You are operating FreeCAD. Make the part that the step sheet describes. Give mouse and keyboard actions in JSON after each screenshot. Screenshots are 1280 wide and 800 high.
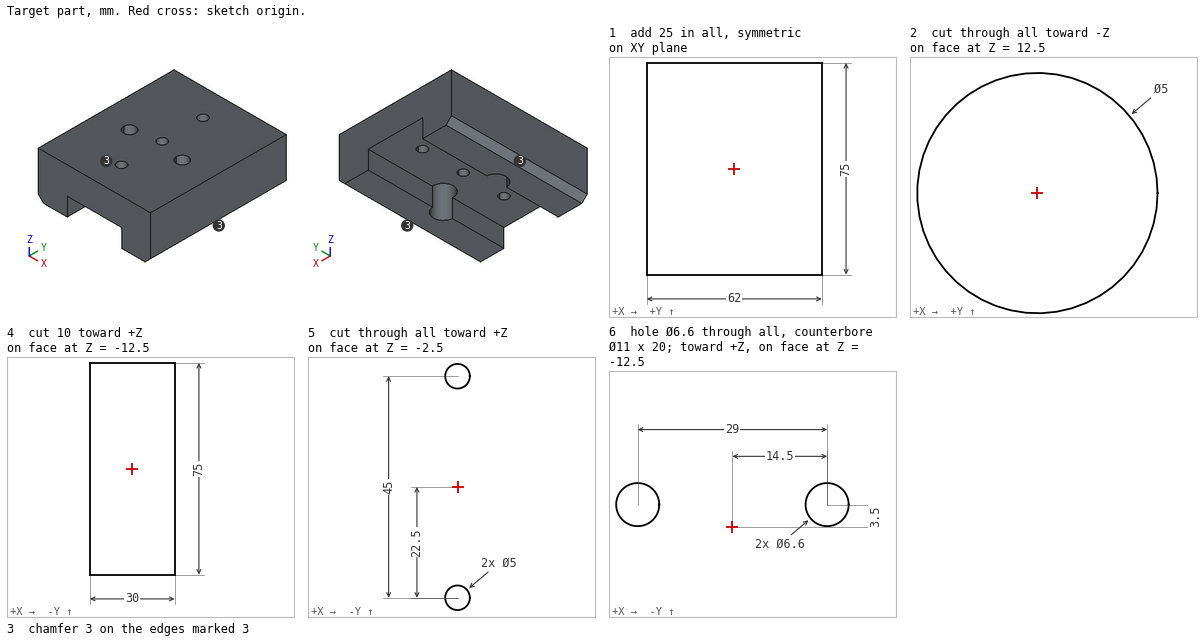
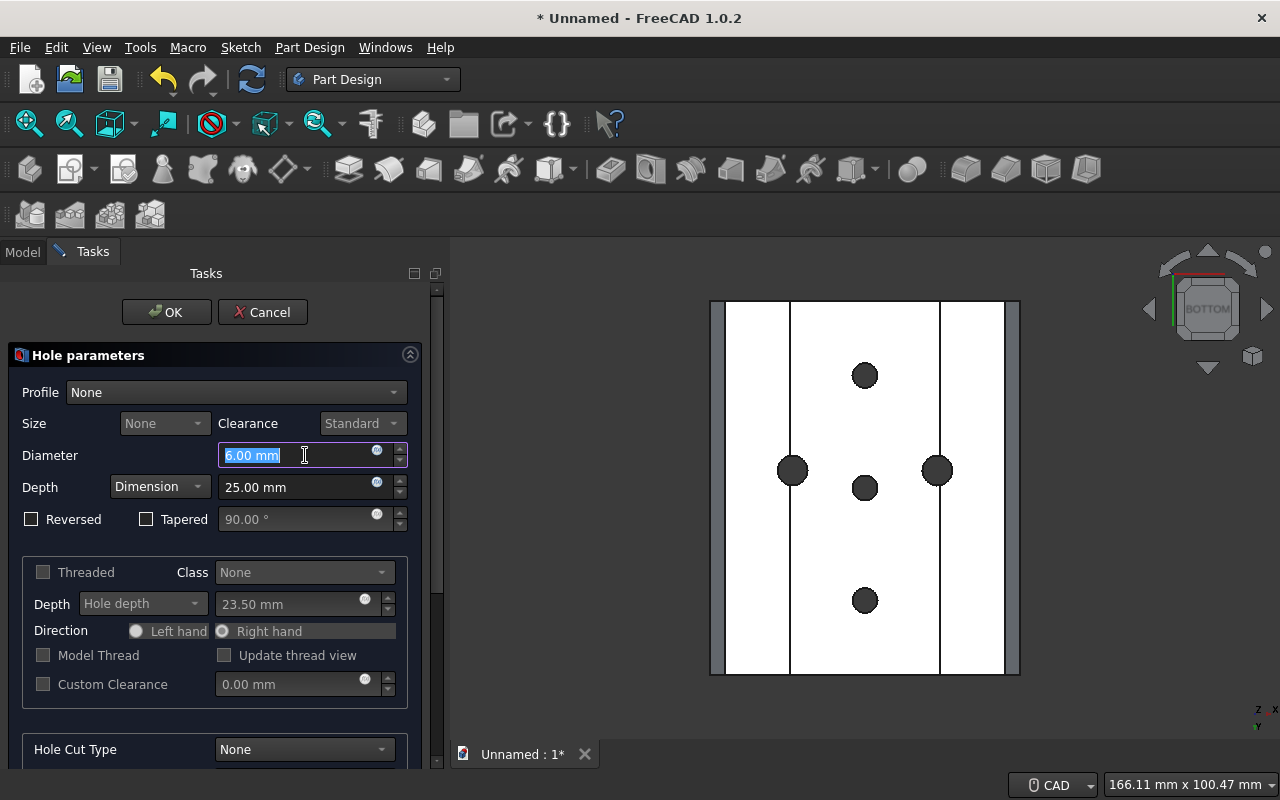
{"action": "type", "text": "6.6"}
{"action": "key", "text": "Tab"}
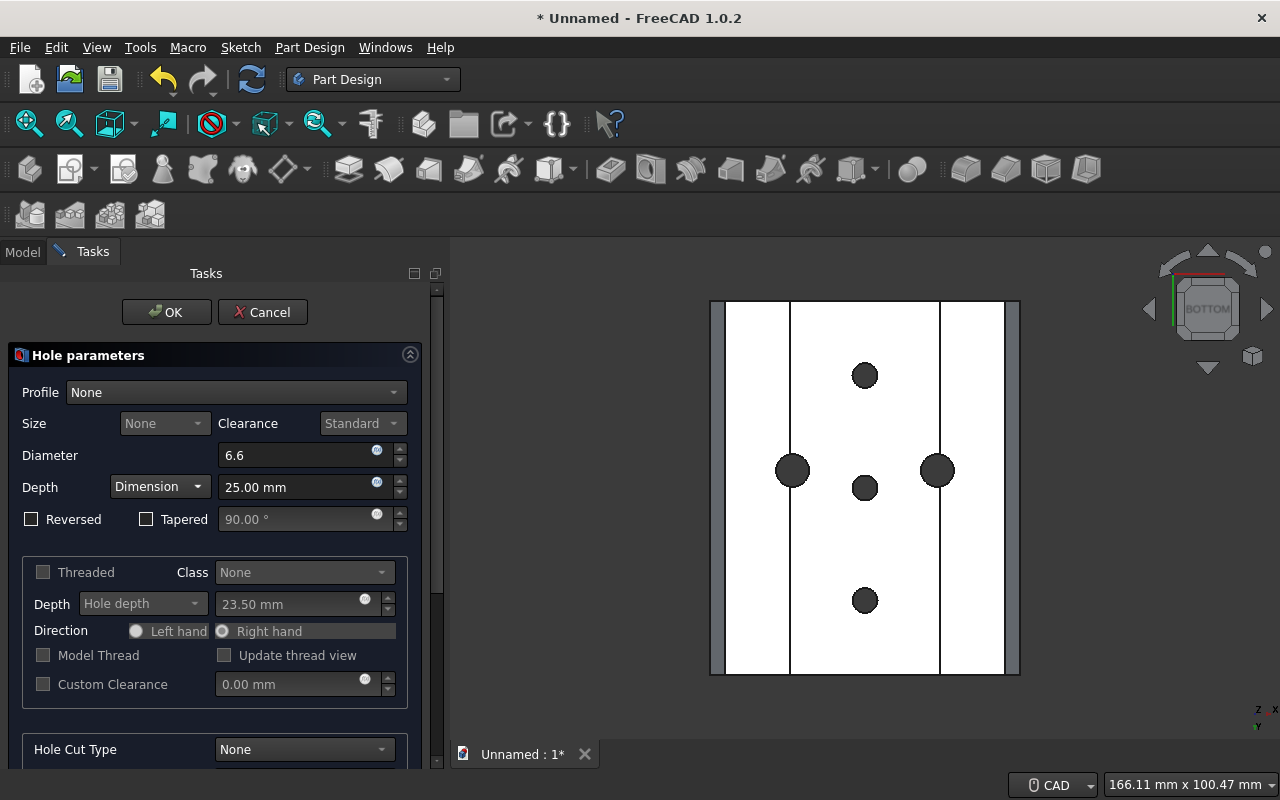
{"action": "left_click", "coordinate": [161, 486]}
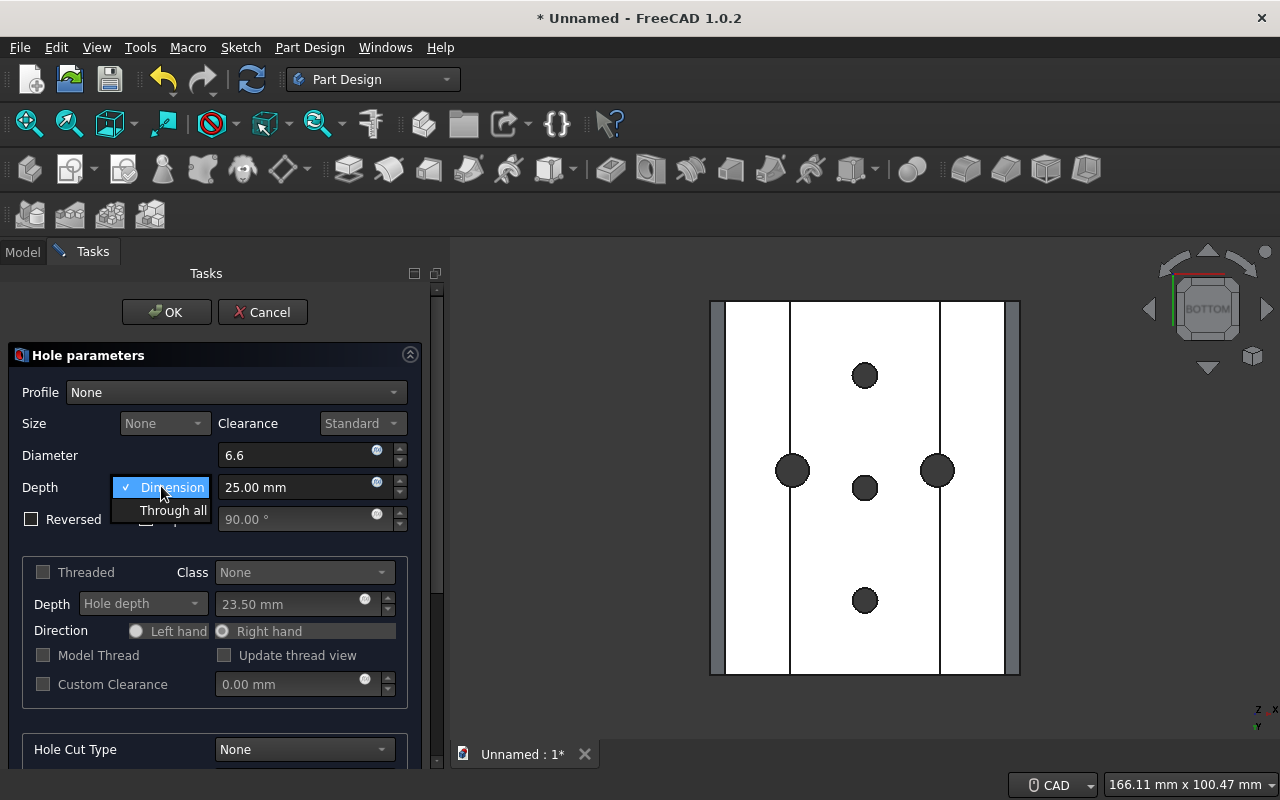
{"action": "left_click", "coordinate": [160, 510]}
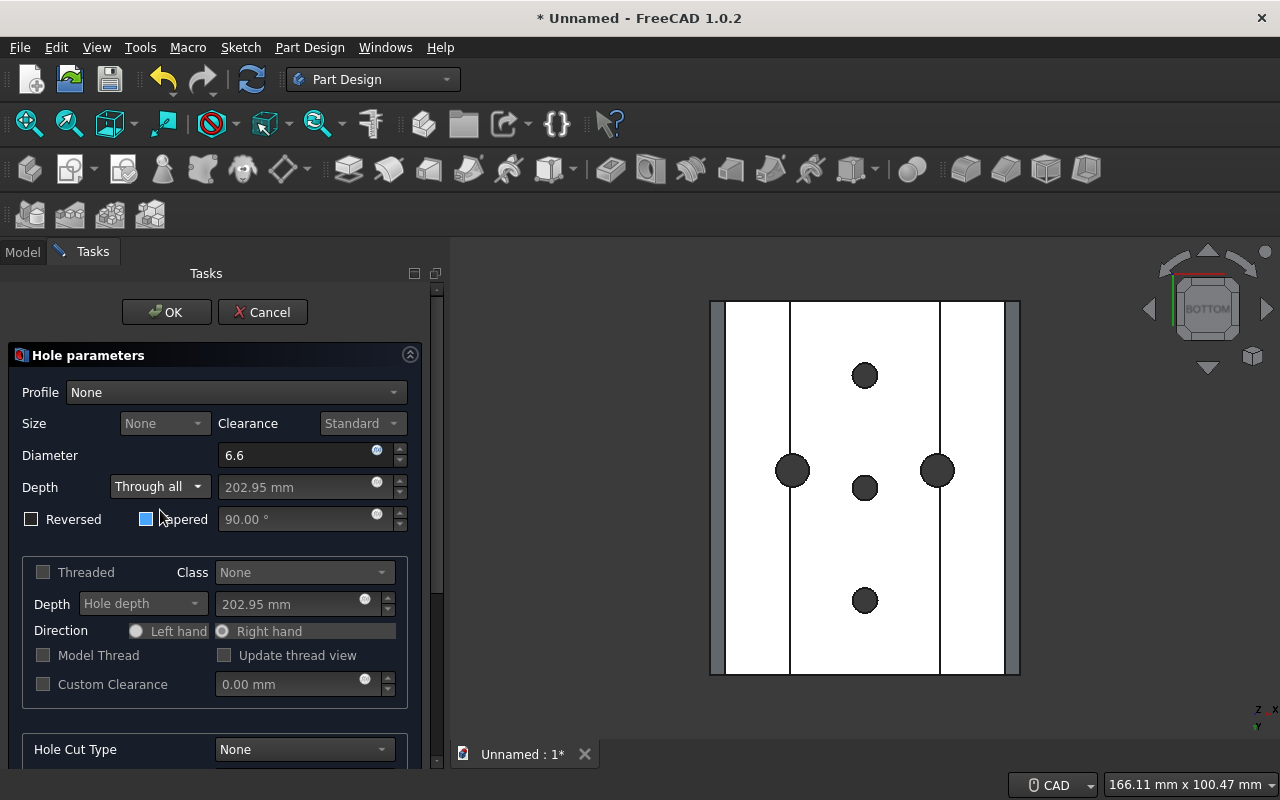
{"action": "left_click", "coordinate": [306, 750]}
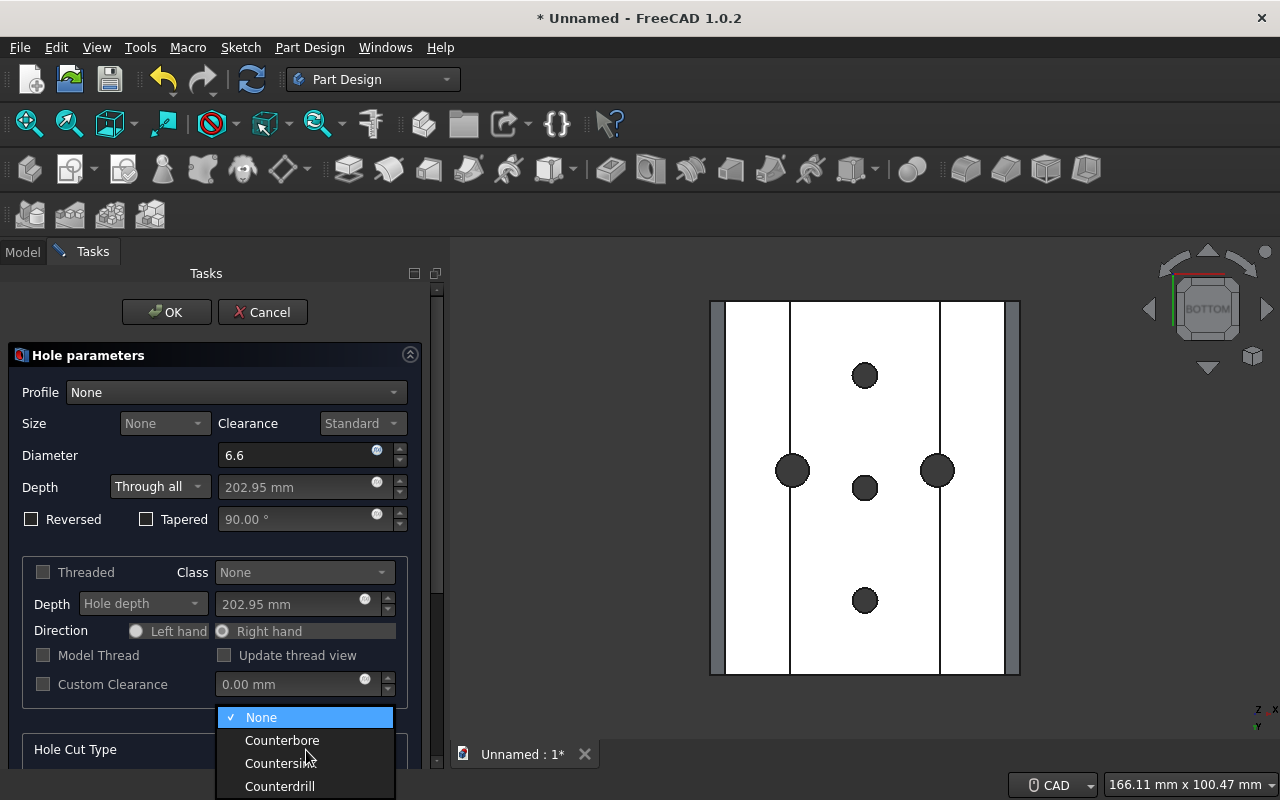
{"action": "left_click", "coordinate": [304, 740]}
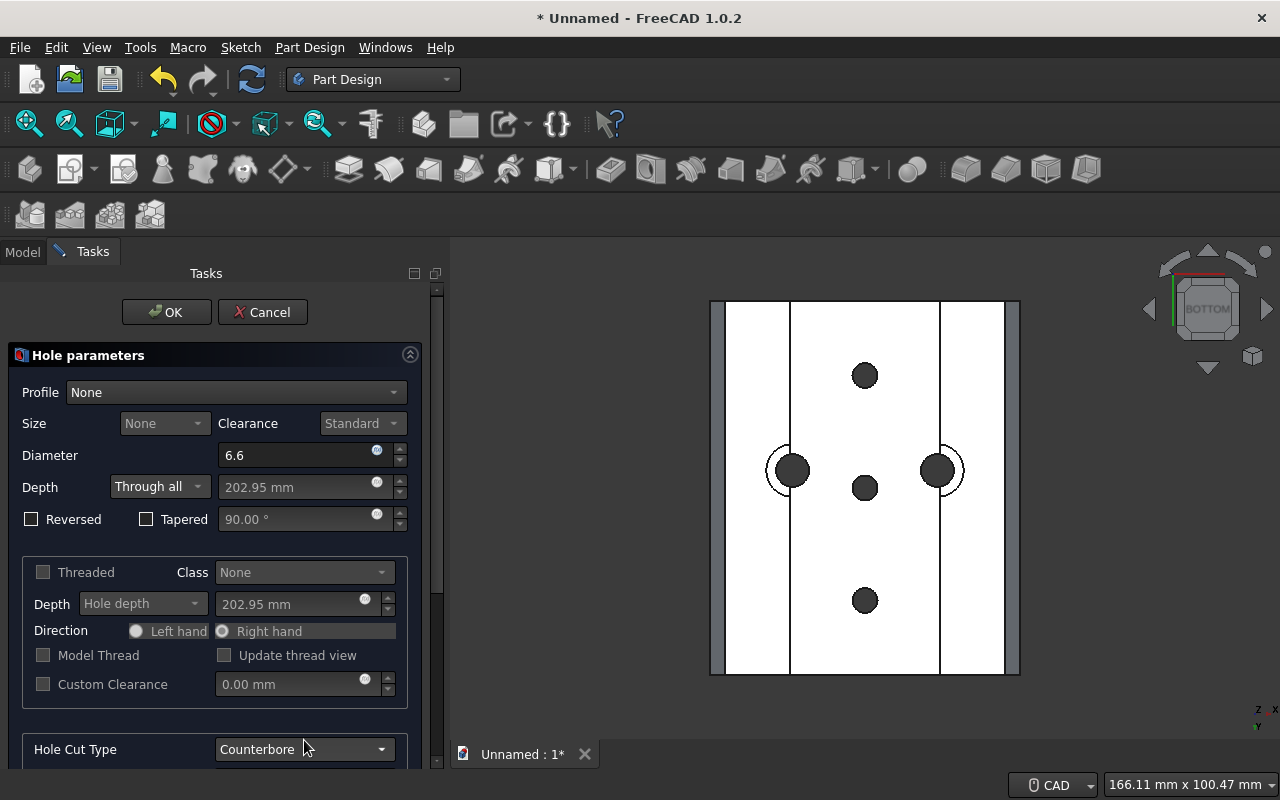
{"action": "scroll", "coordinate": [437, 526], "scroll_direction": "down", "scroll_amount": 2}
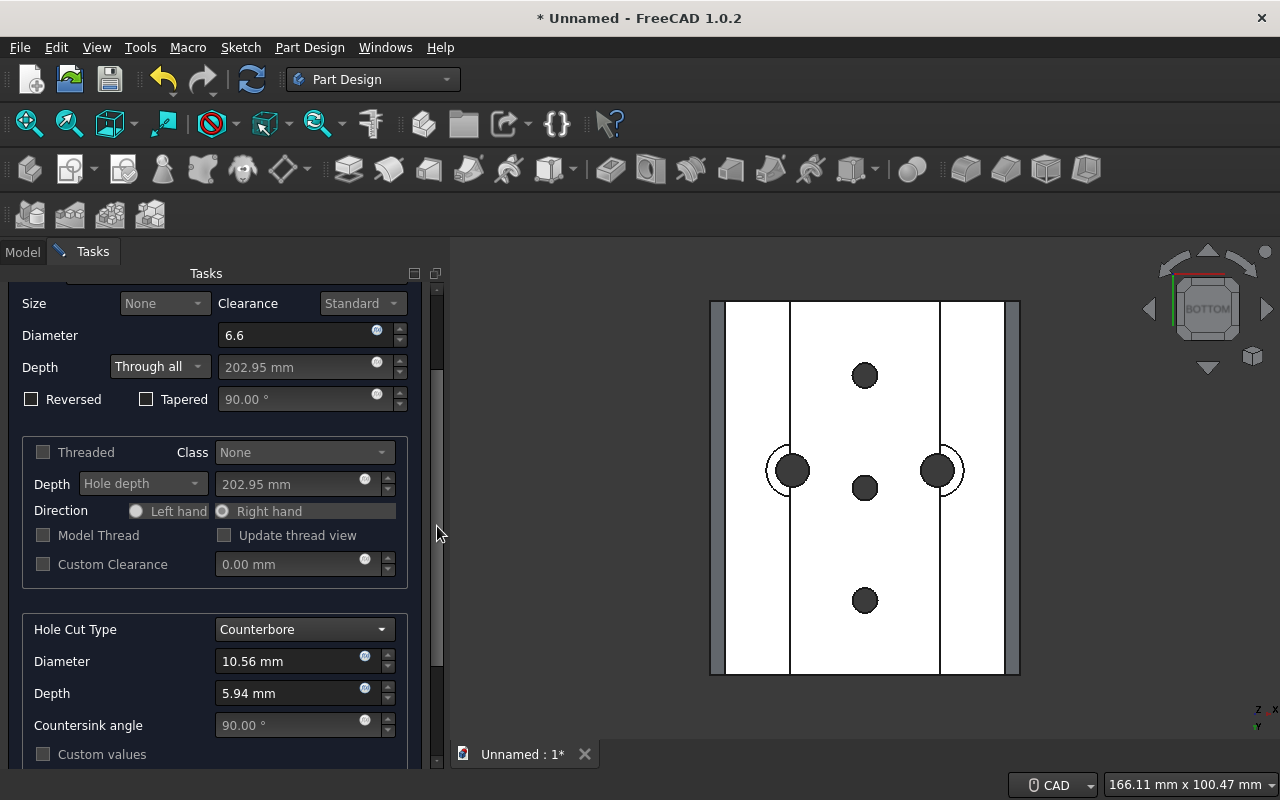
{"action": "triple_click", "coordinate": [298, 661]}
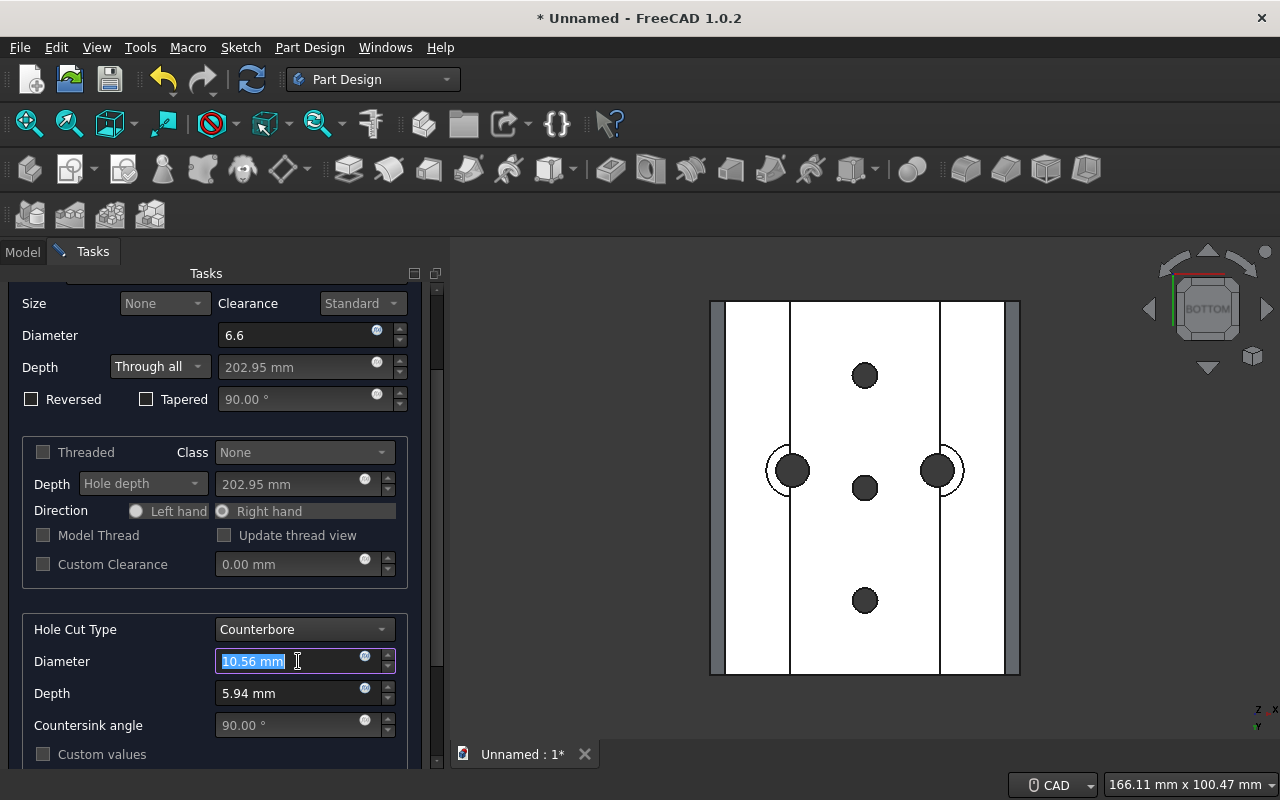
{"action": "type", "text": "11"}
{"action": "key", "text": "Tab"}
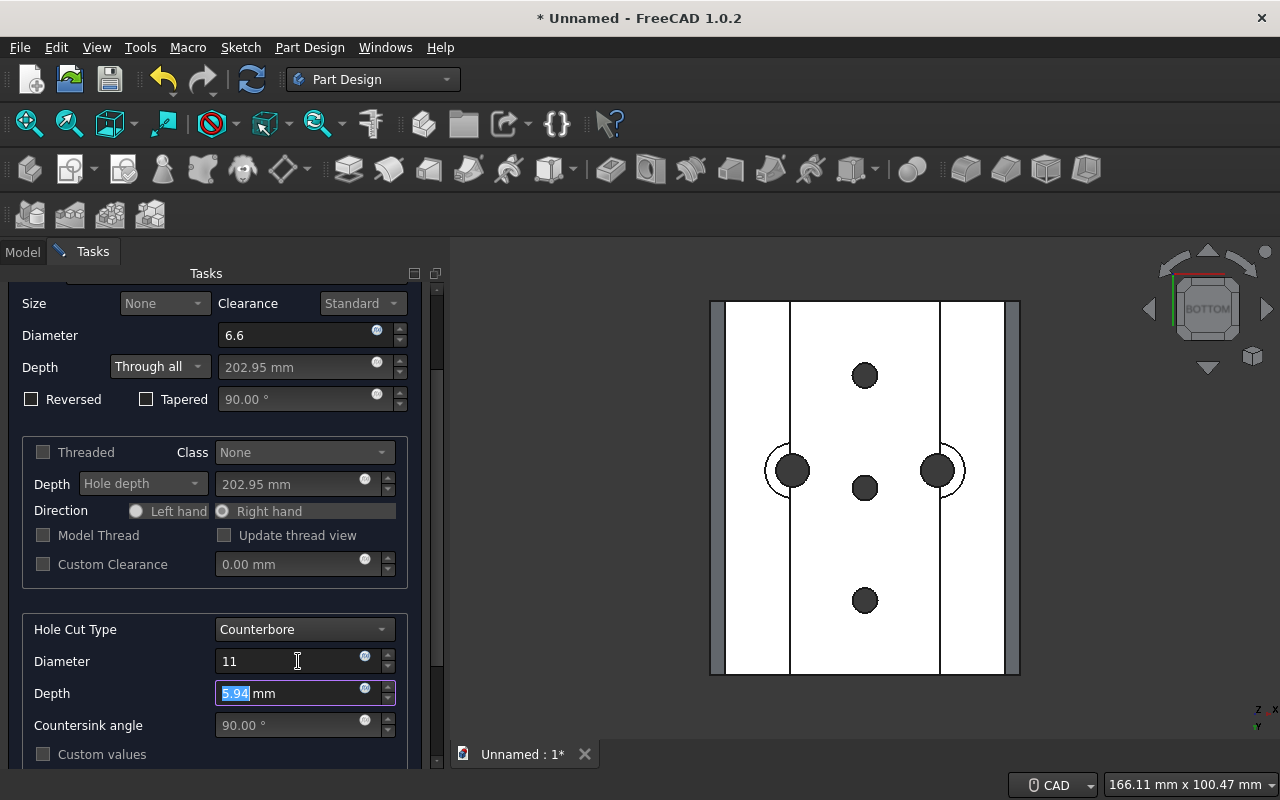
{"action": "type", "text": "20"}
{"action": "key", "text": "Tab"}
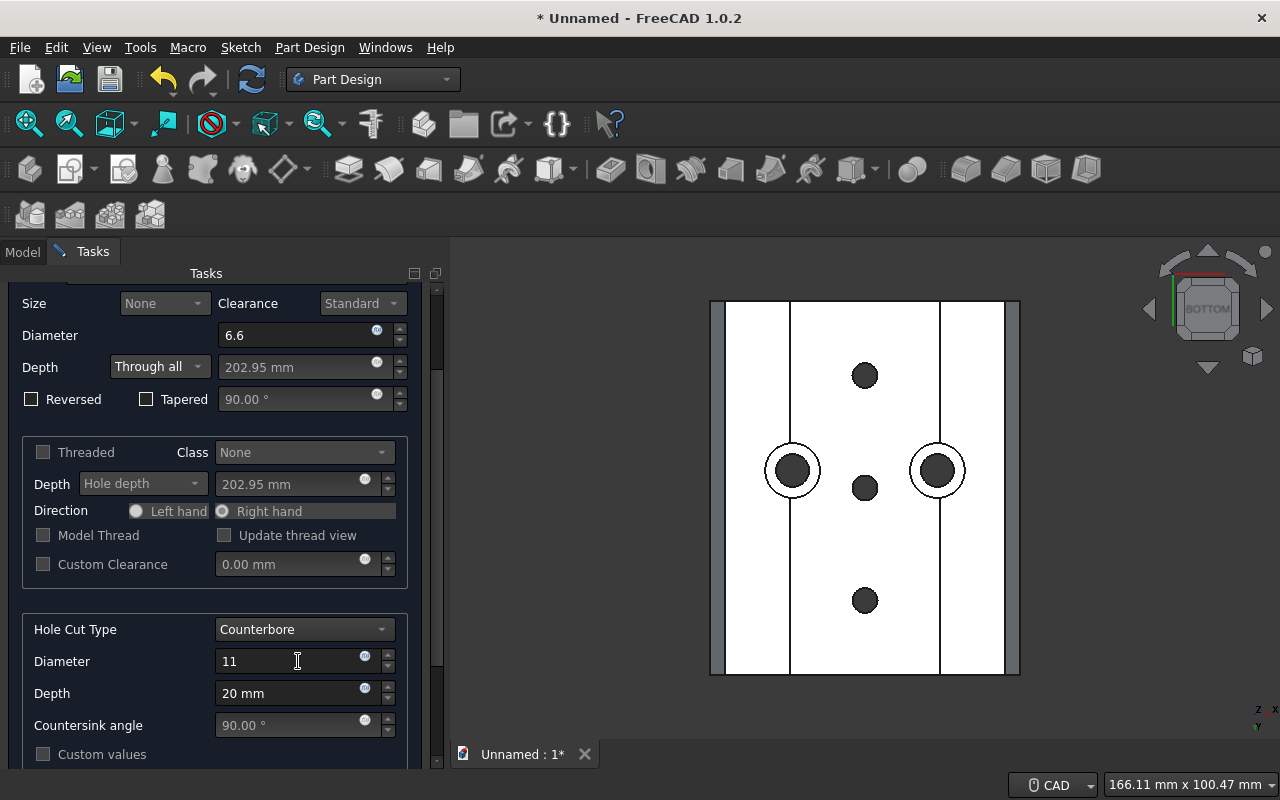
{"action": "scroll", "coordinate": [437, 526], "scroll_direction": "up", "scroll_amount": 3}